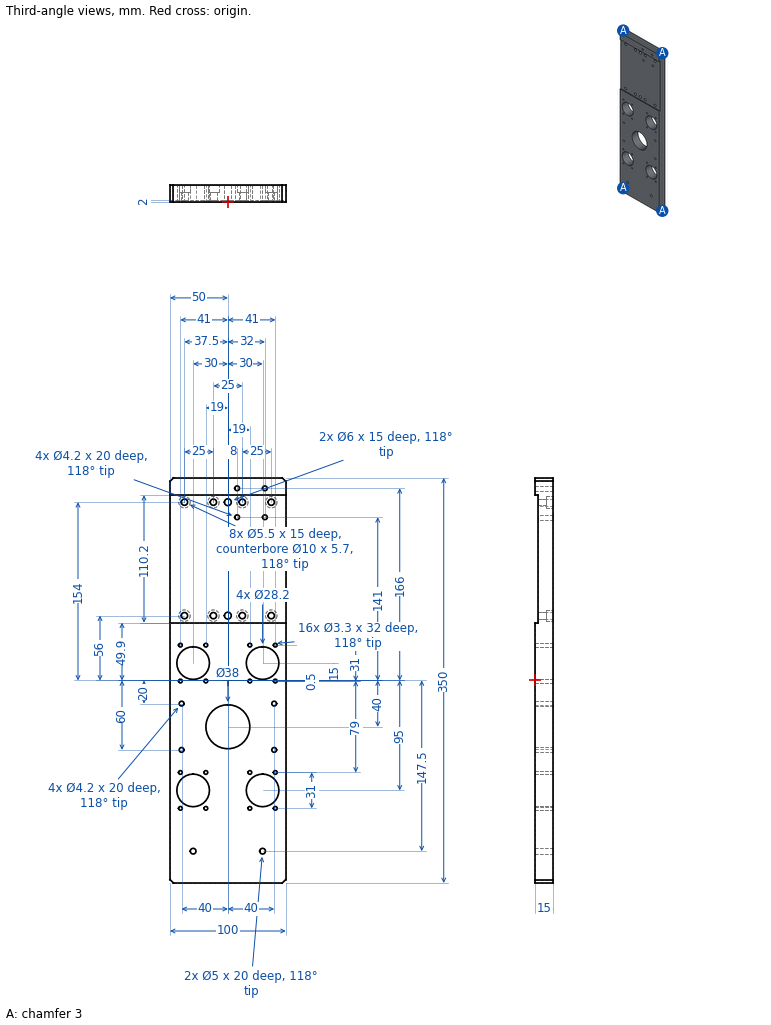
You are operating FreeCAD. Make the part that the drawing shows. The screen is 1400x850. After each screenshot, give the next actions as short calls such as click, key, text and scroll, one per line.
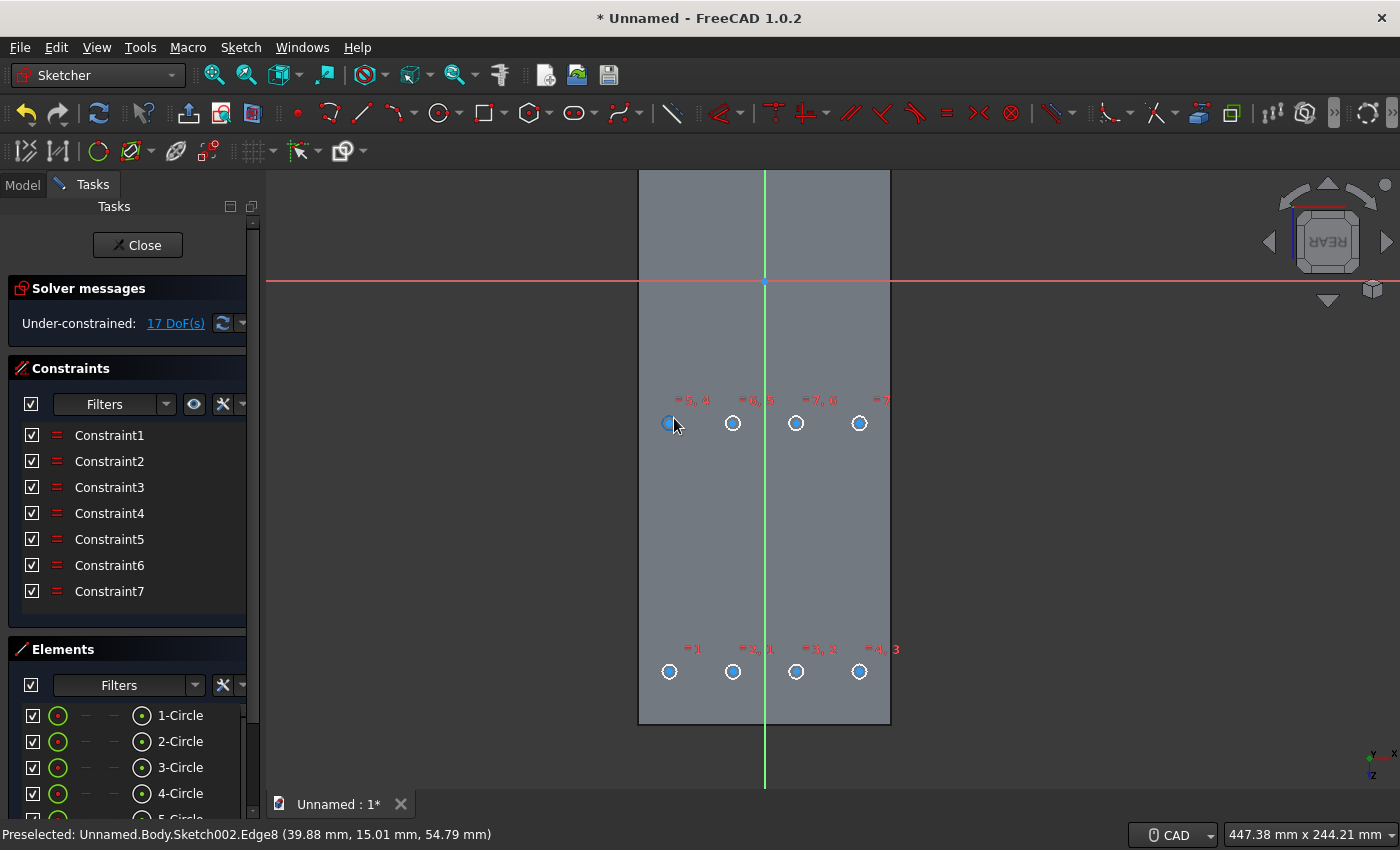
click(669, 672)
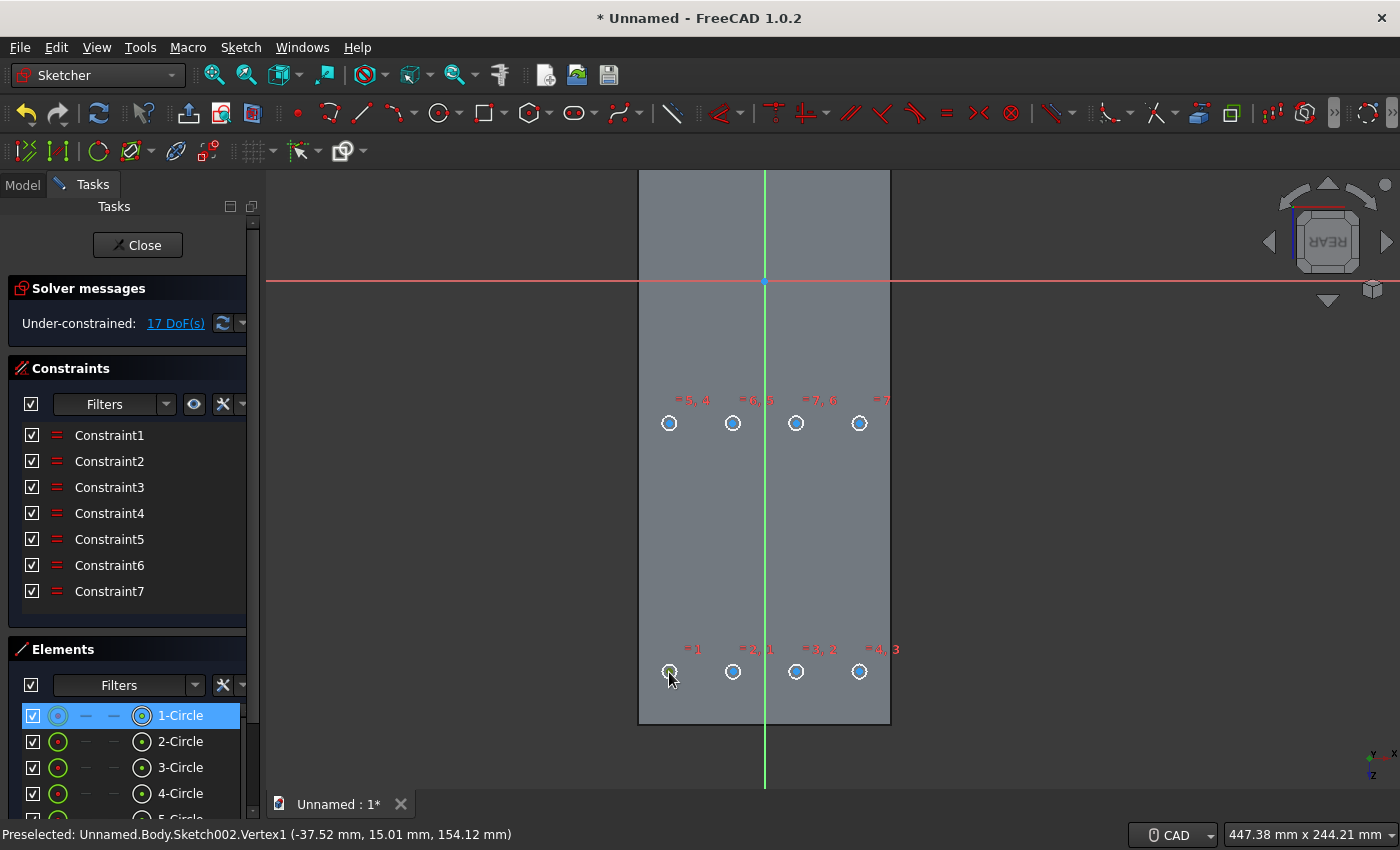
click(733, 672)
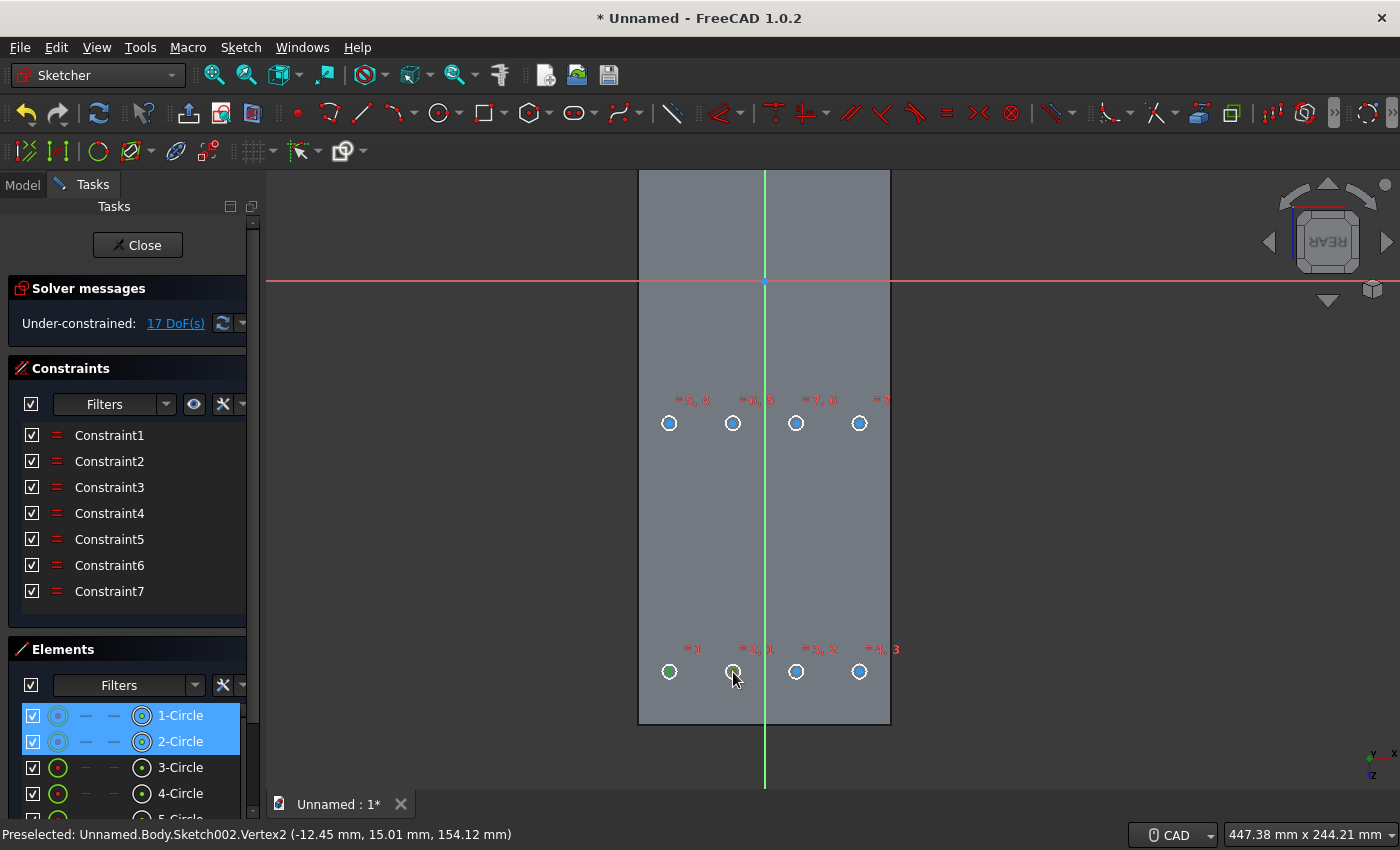
key(h)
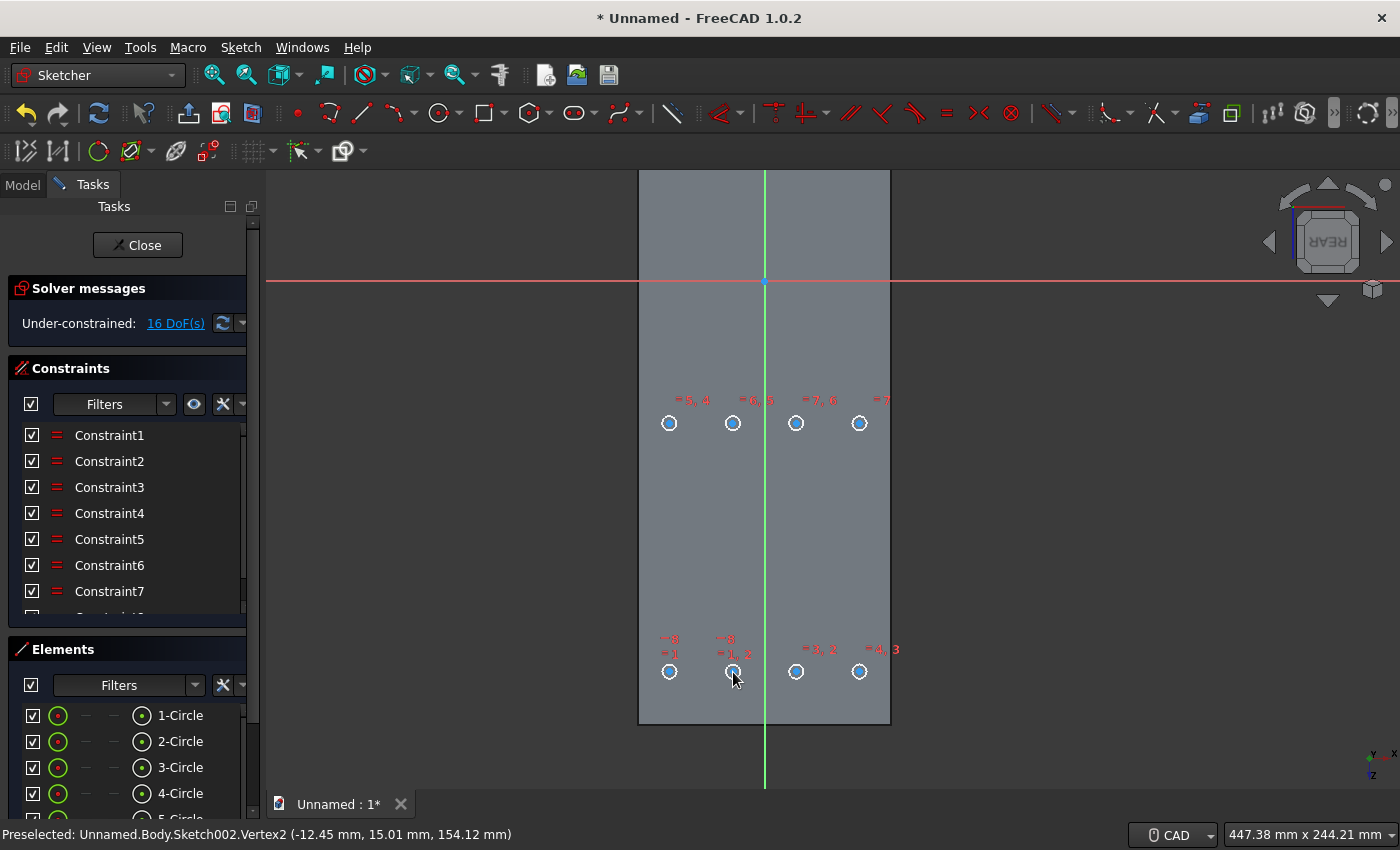
click(733, 672)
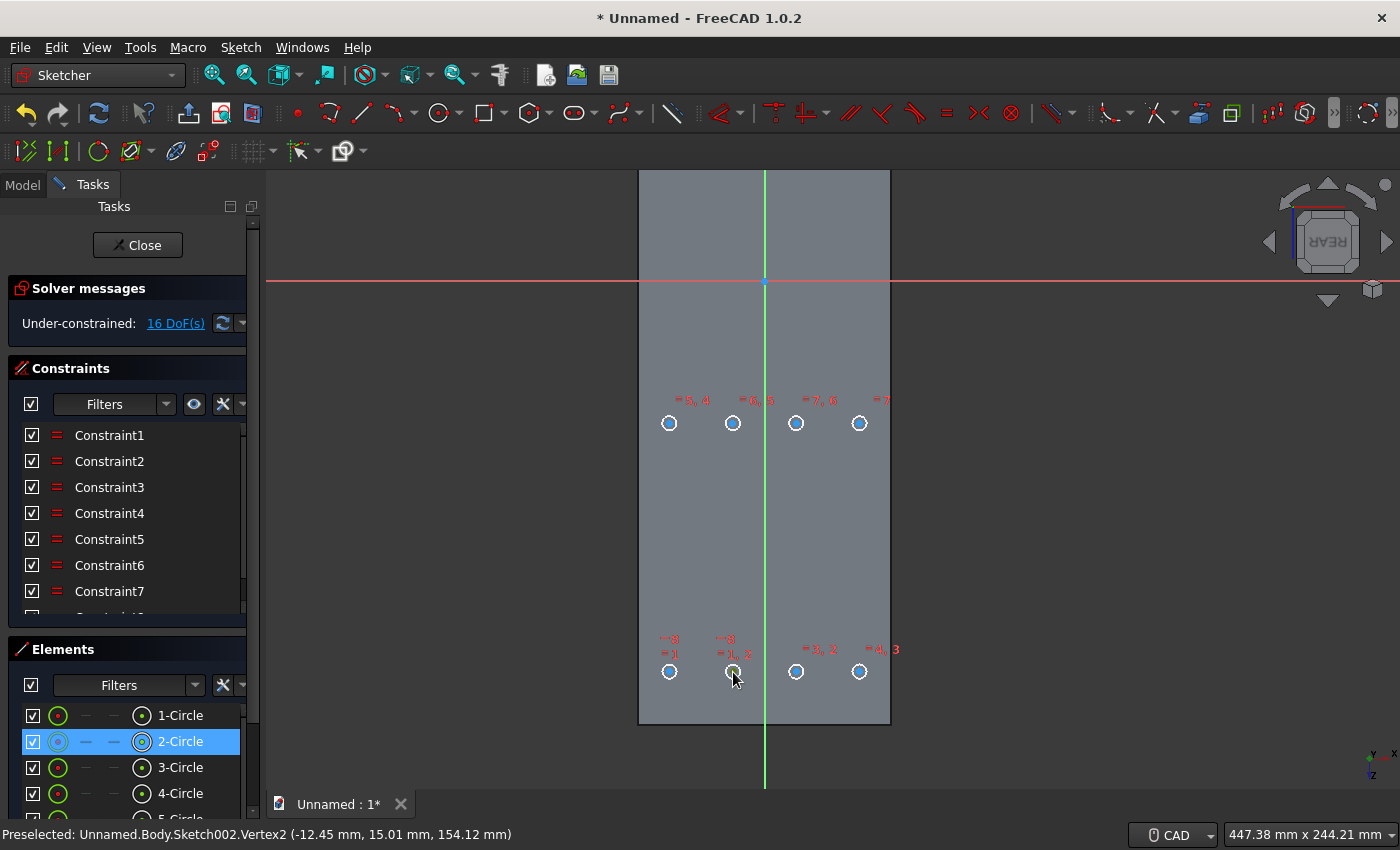
click(796, 672)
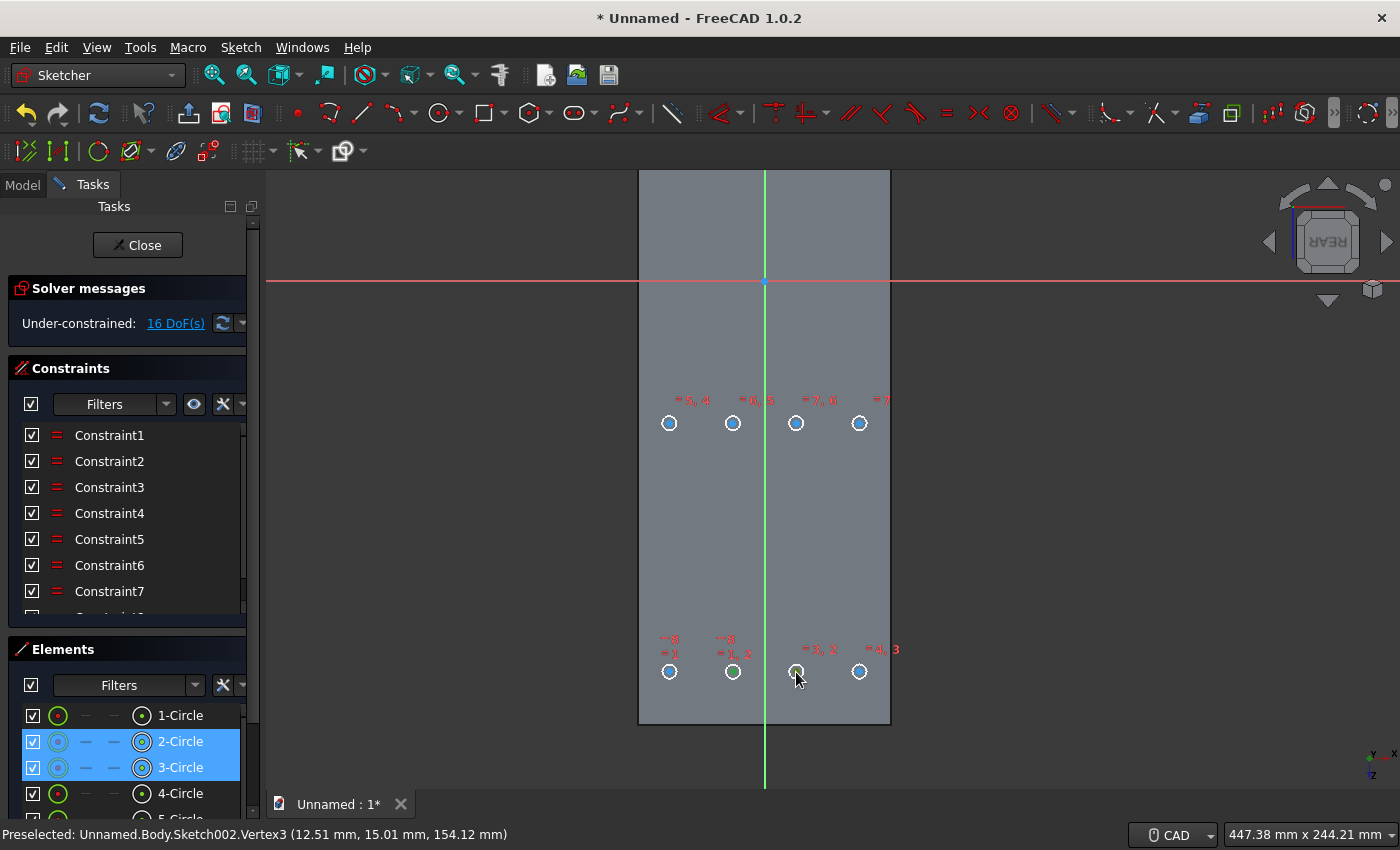
click(828, 114)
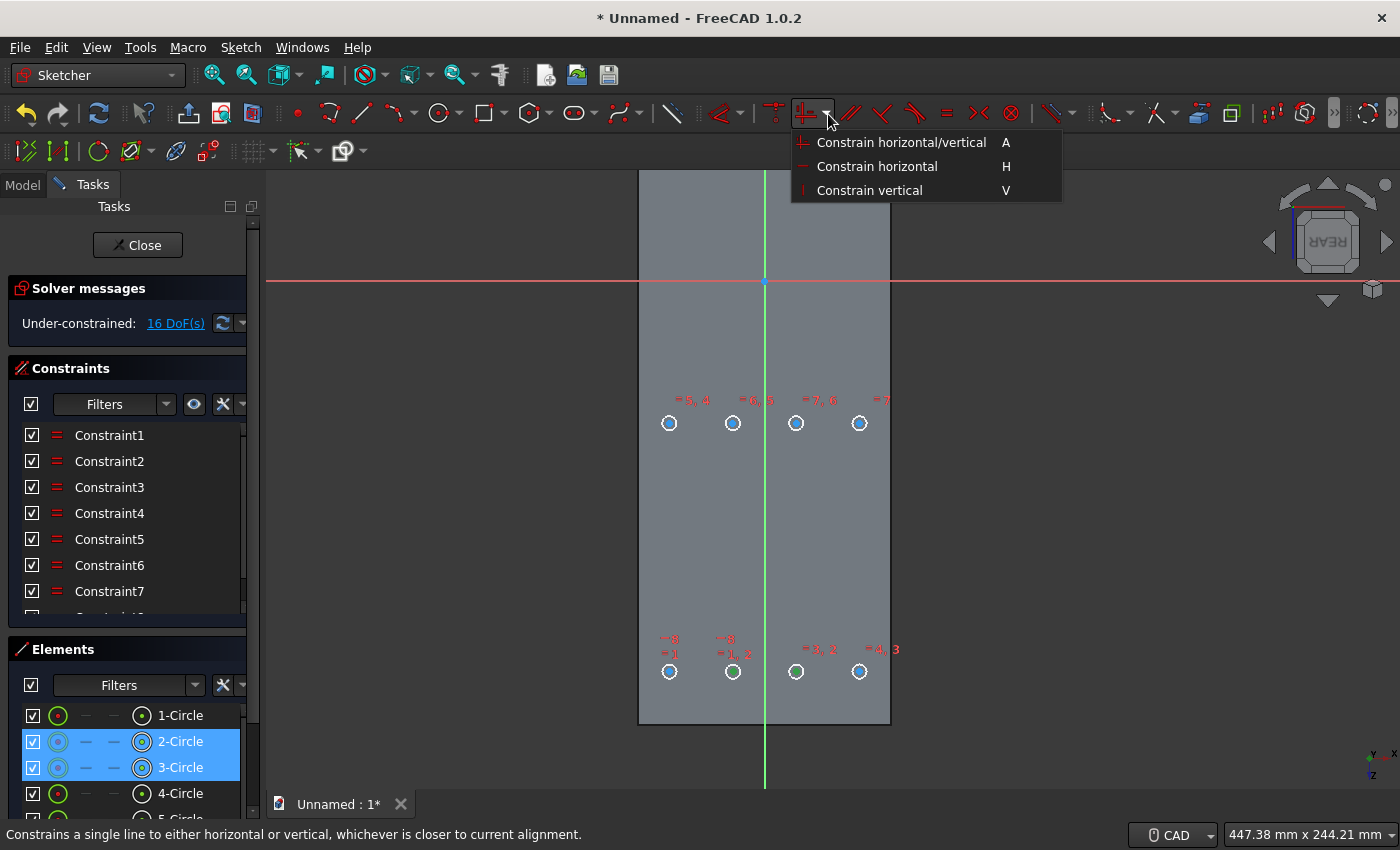
click(927, 166)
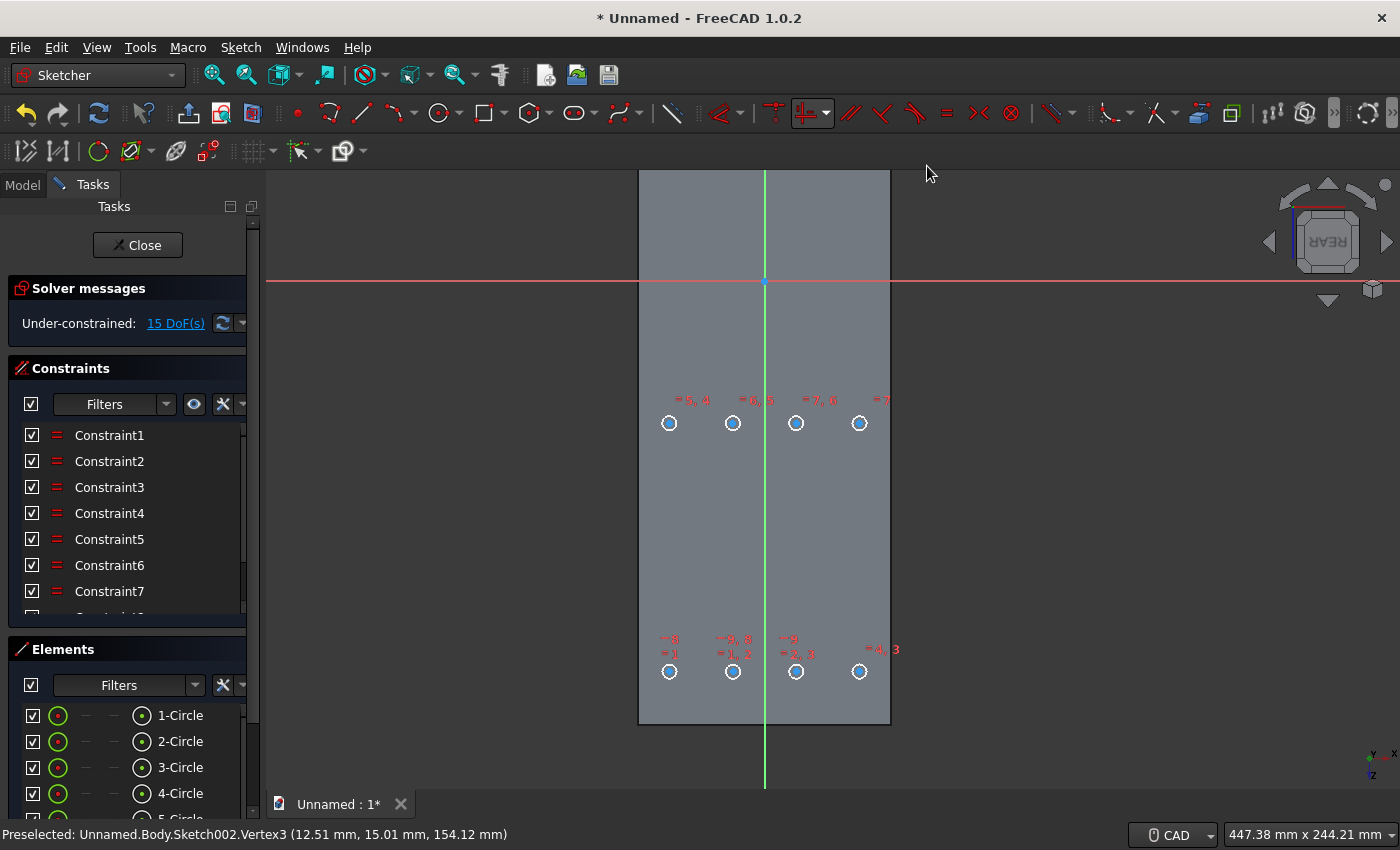
click(796, 672)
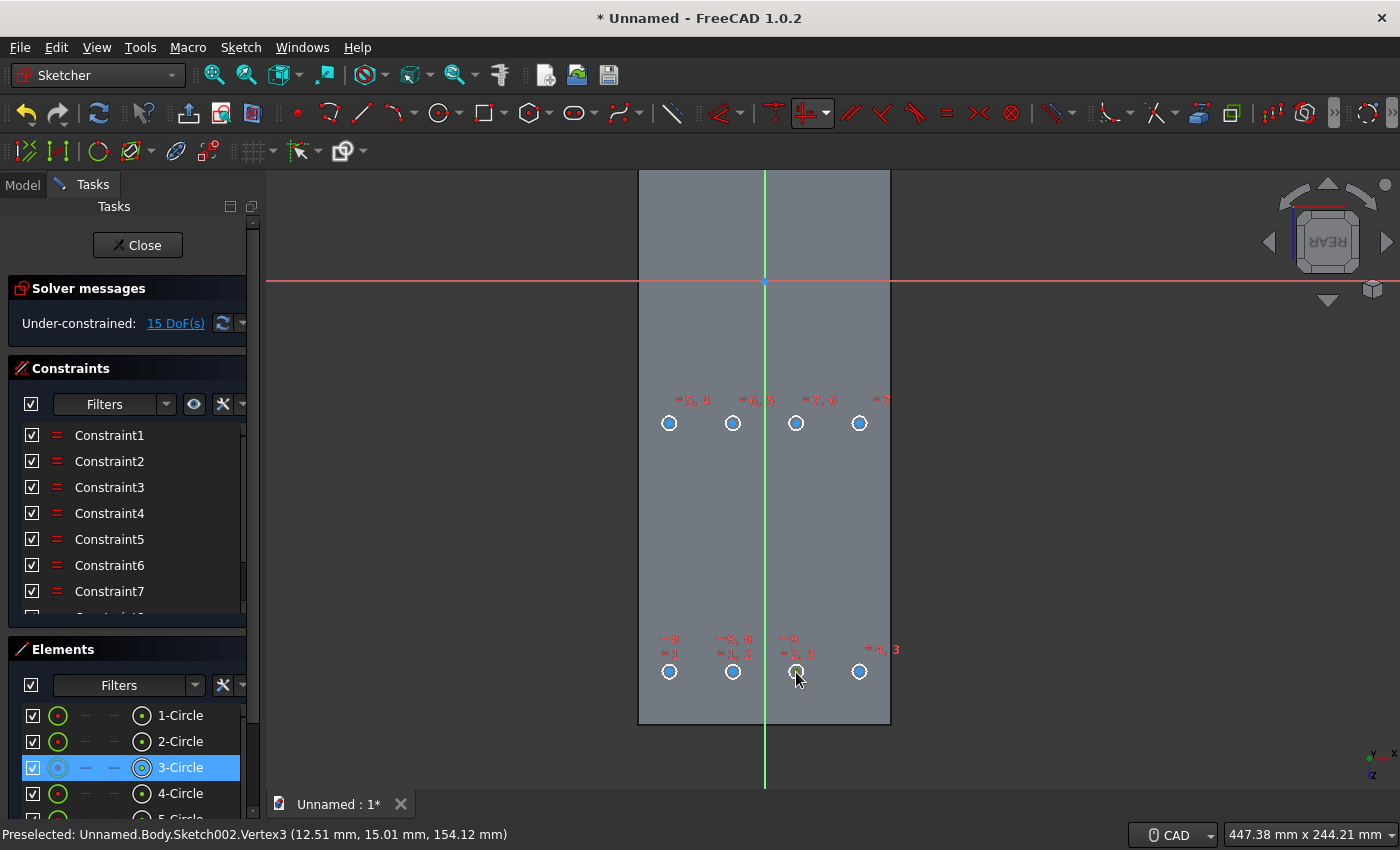
click(860, 672)